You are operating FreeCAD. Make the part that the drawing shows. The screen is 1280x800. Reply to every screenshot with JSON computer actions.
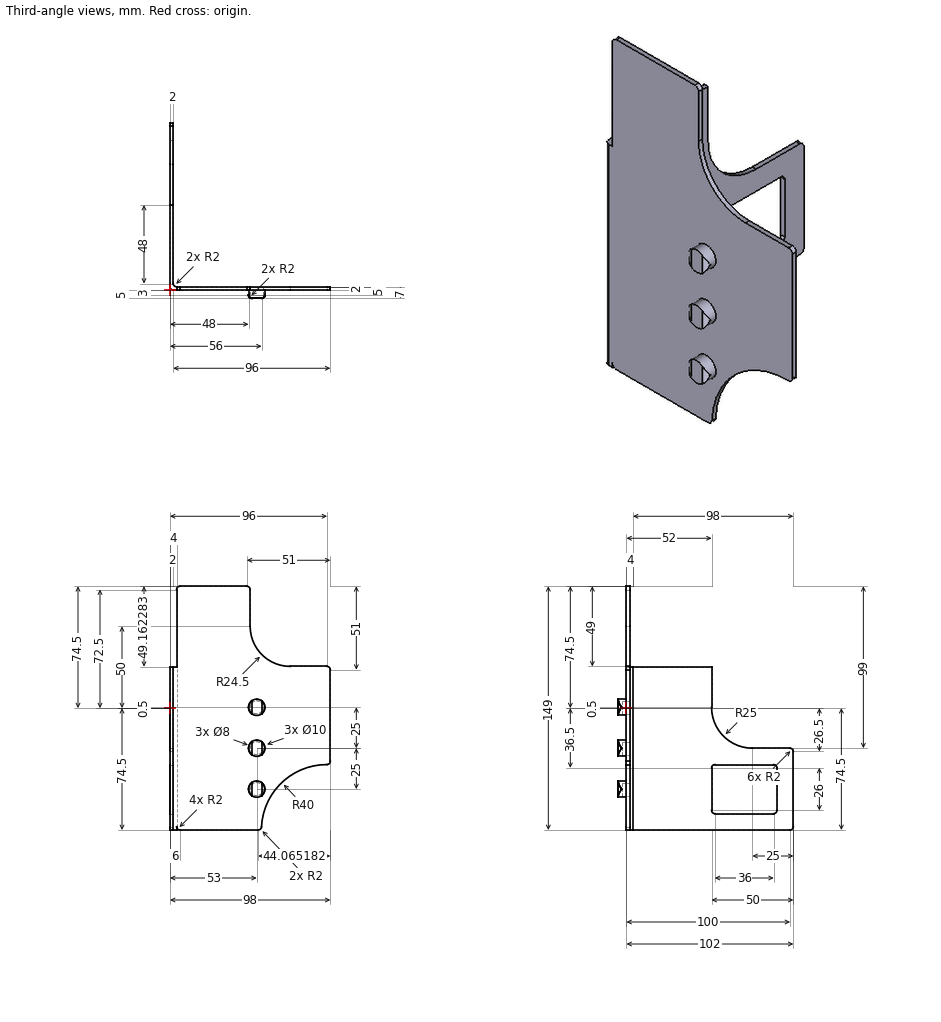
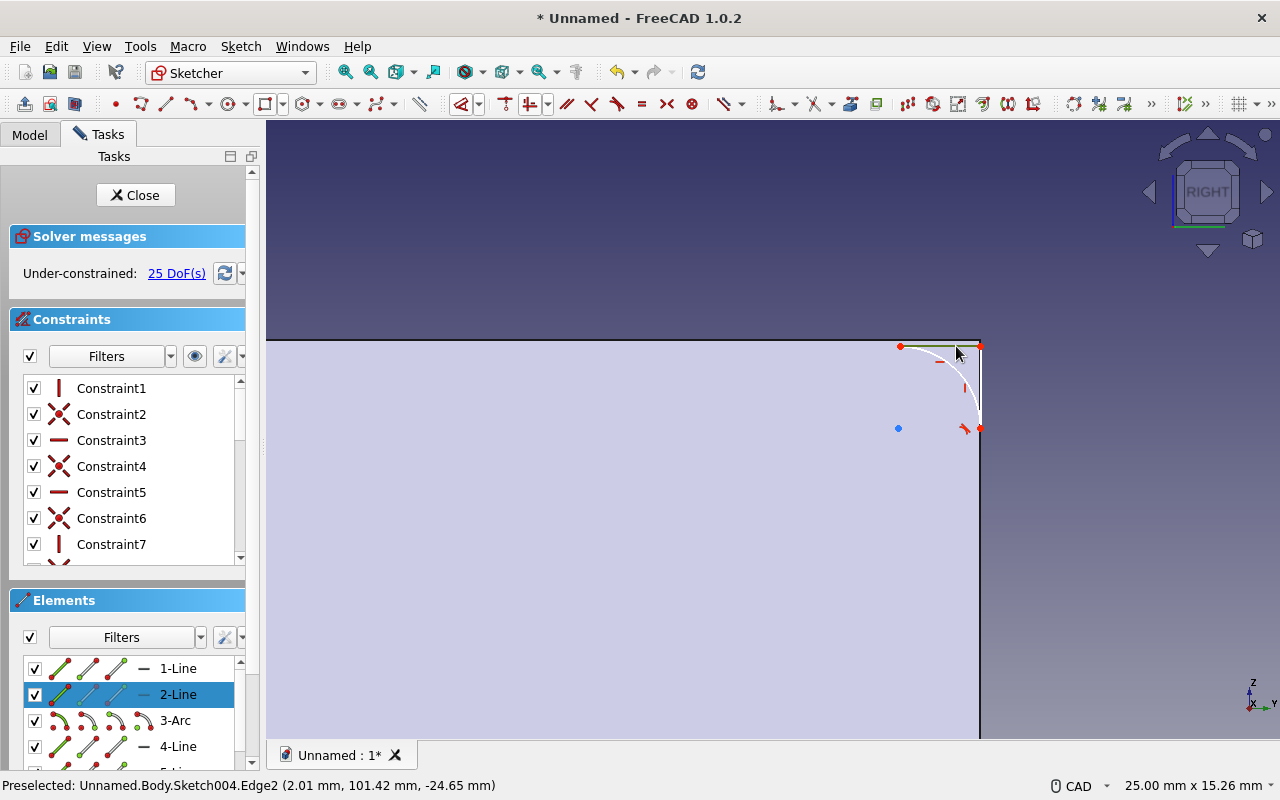
{"action": "scroll", "coordinate": [937, 356], "scroll_direction": "up", "scroll_amount": 3}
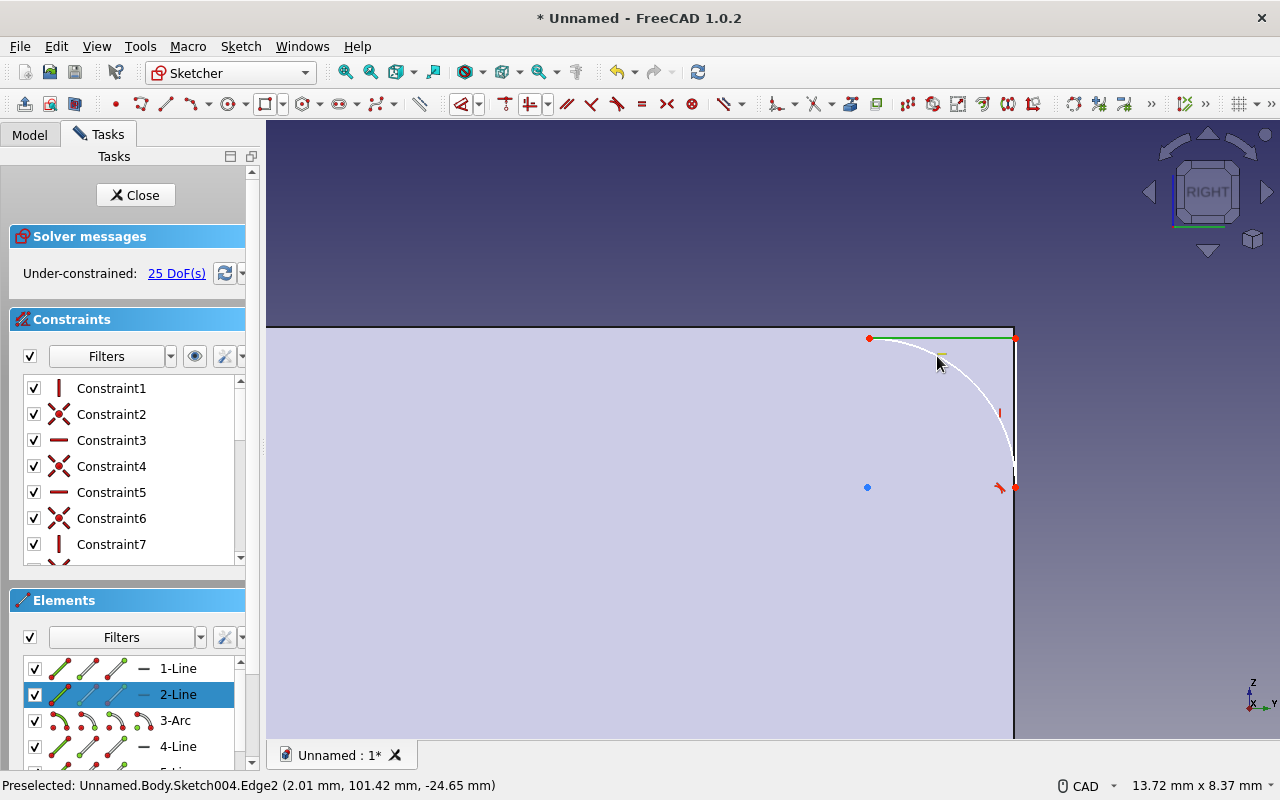
{"action": "left_click", "coordinate": [936, 355]}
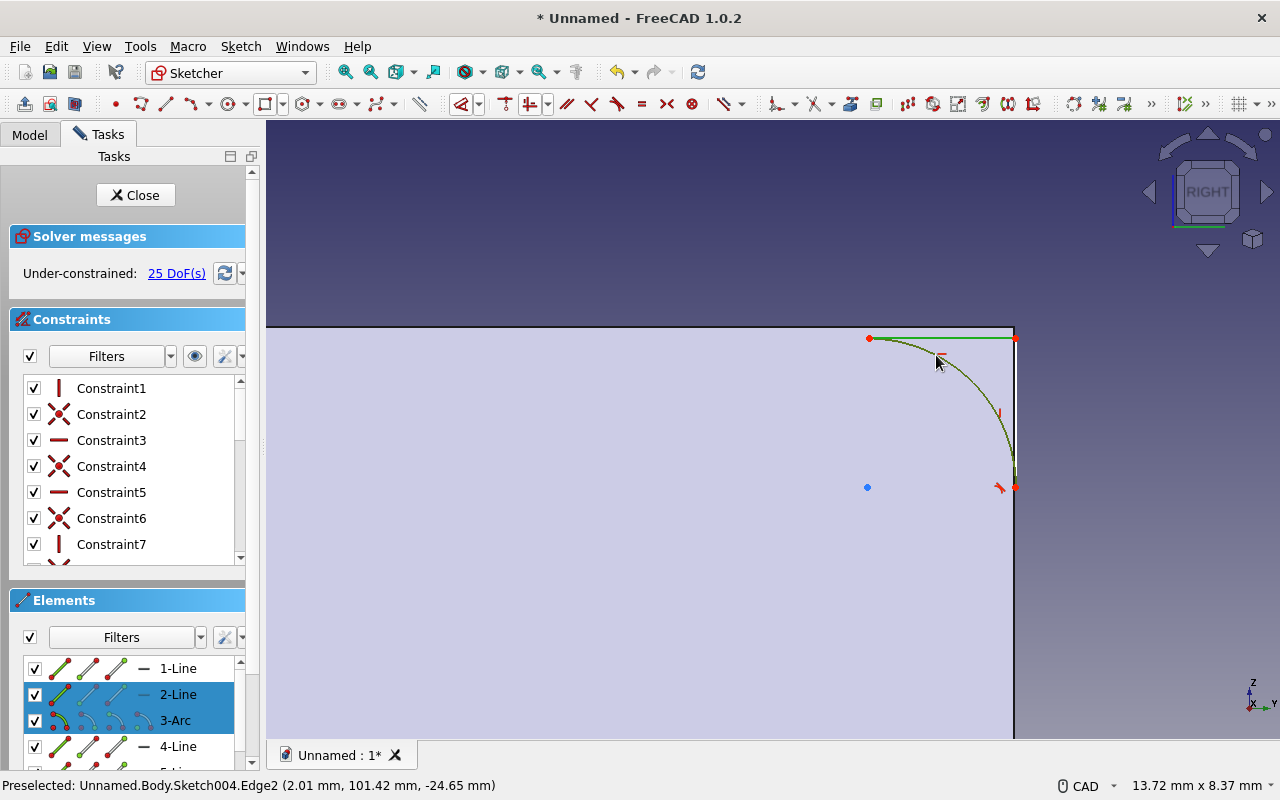
{"action": "key", "text": "t"}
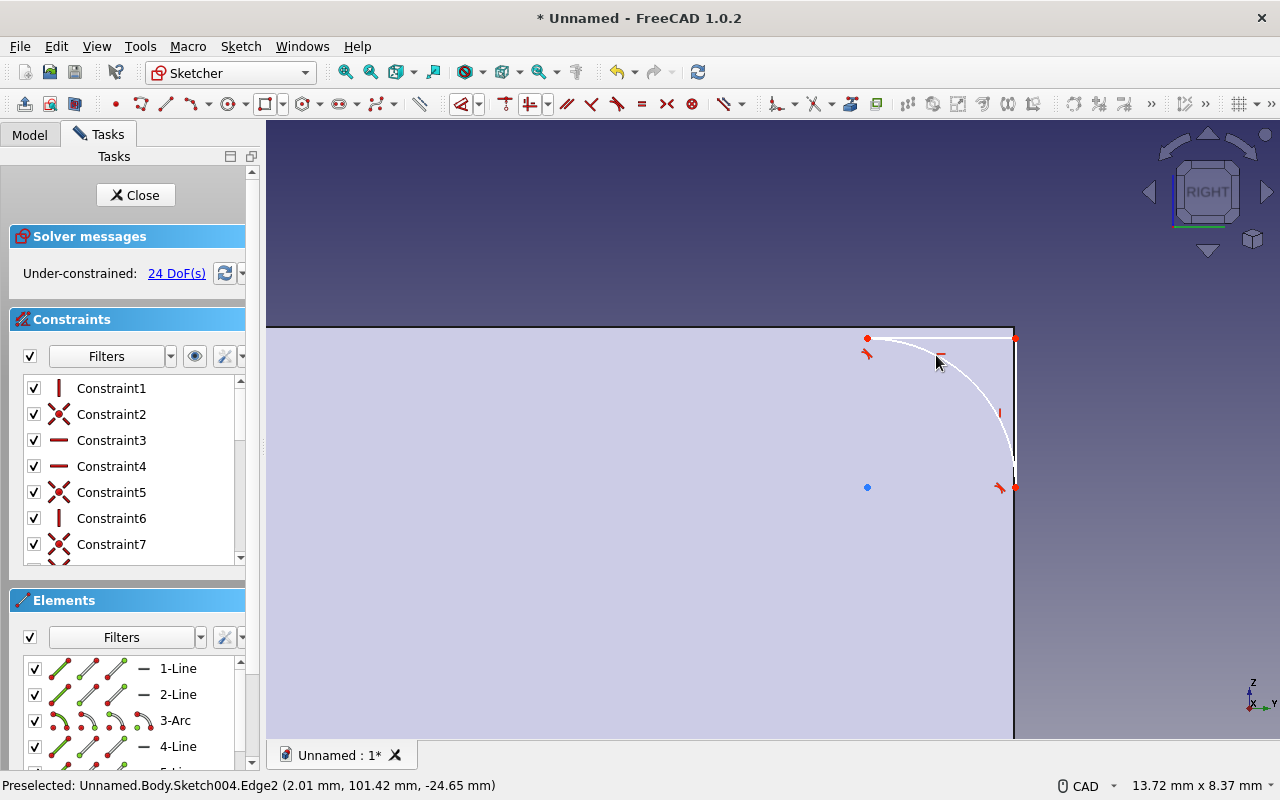
{"action": "scroll", "coordinate": [982, 362], "scroll_direction": "down", "scroll_amount": 13}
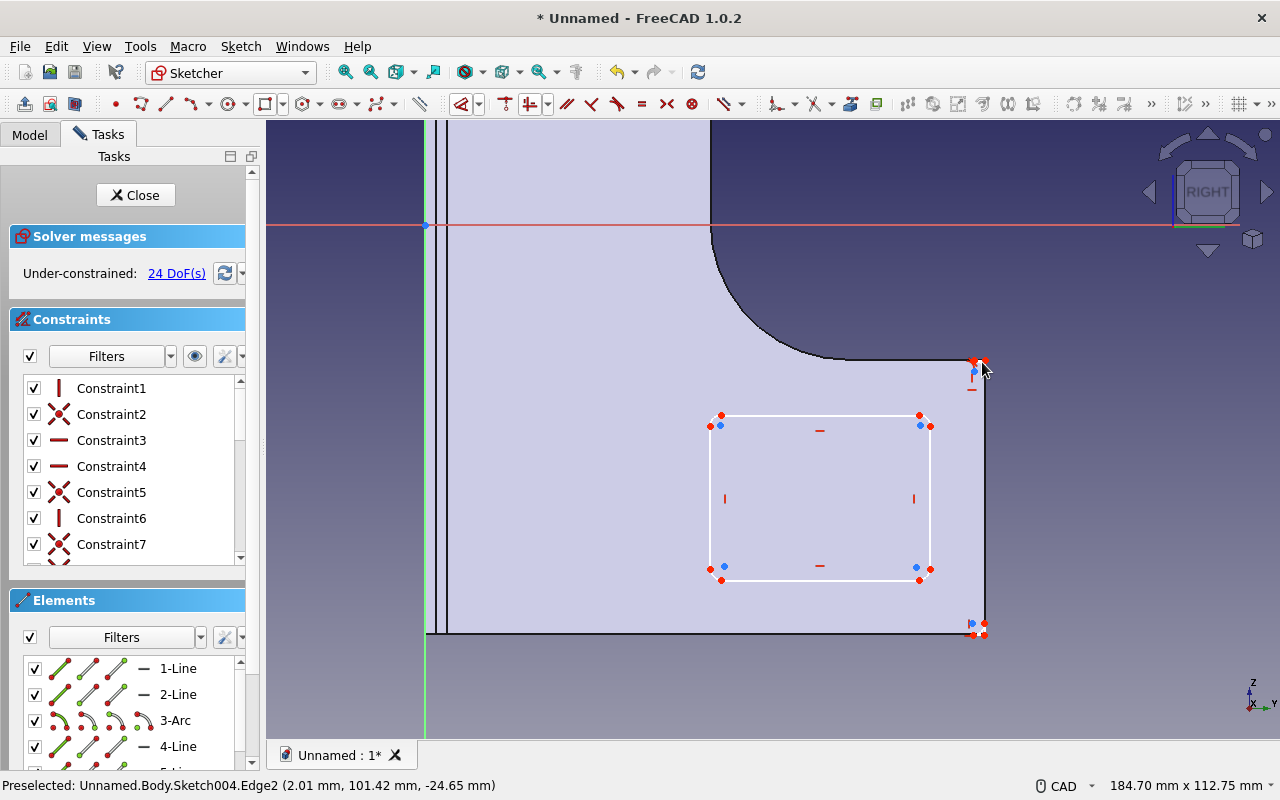
{"action": "scroll", "coordinate": [982, 635], "scroll_direction": "up", "scroll_amount": 9}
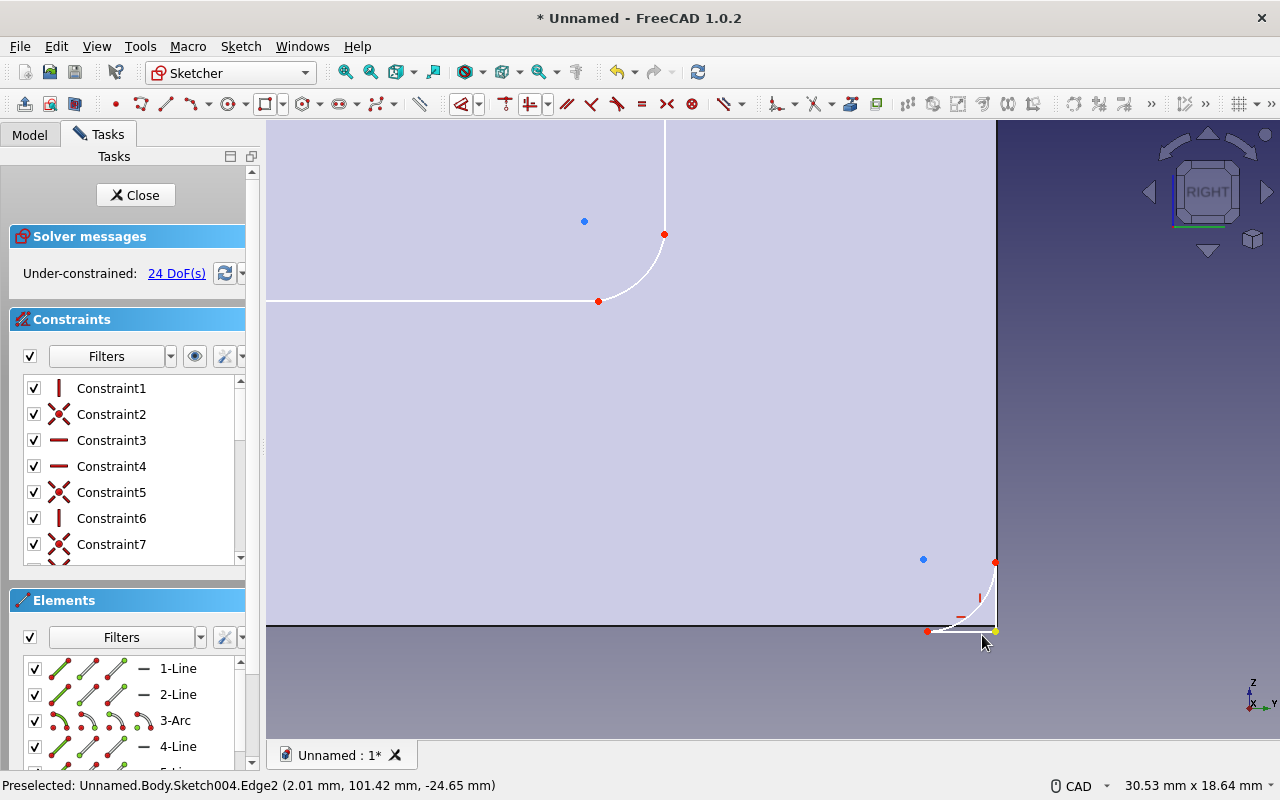
{"action": "left_click", "coordinate": [975, 632]}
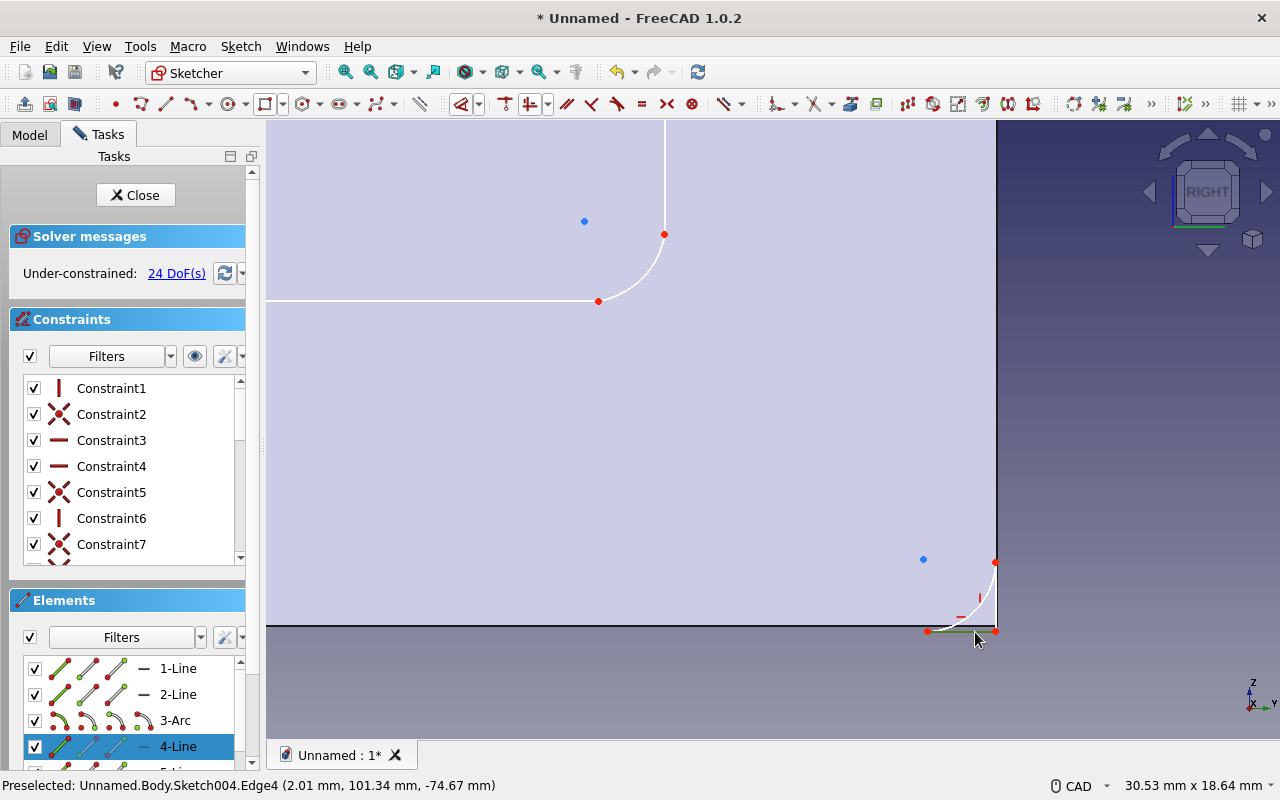
{"action": "left_click", "coordinate": [975, 610]}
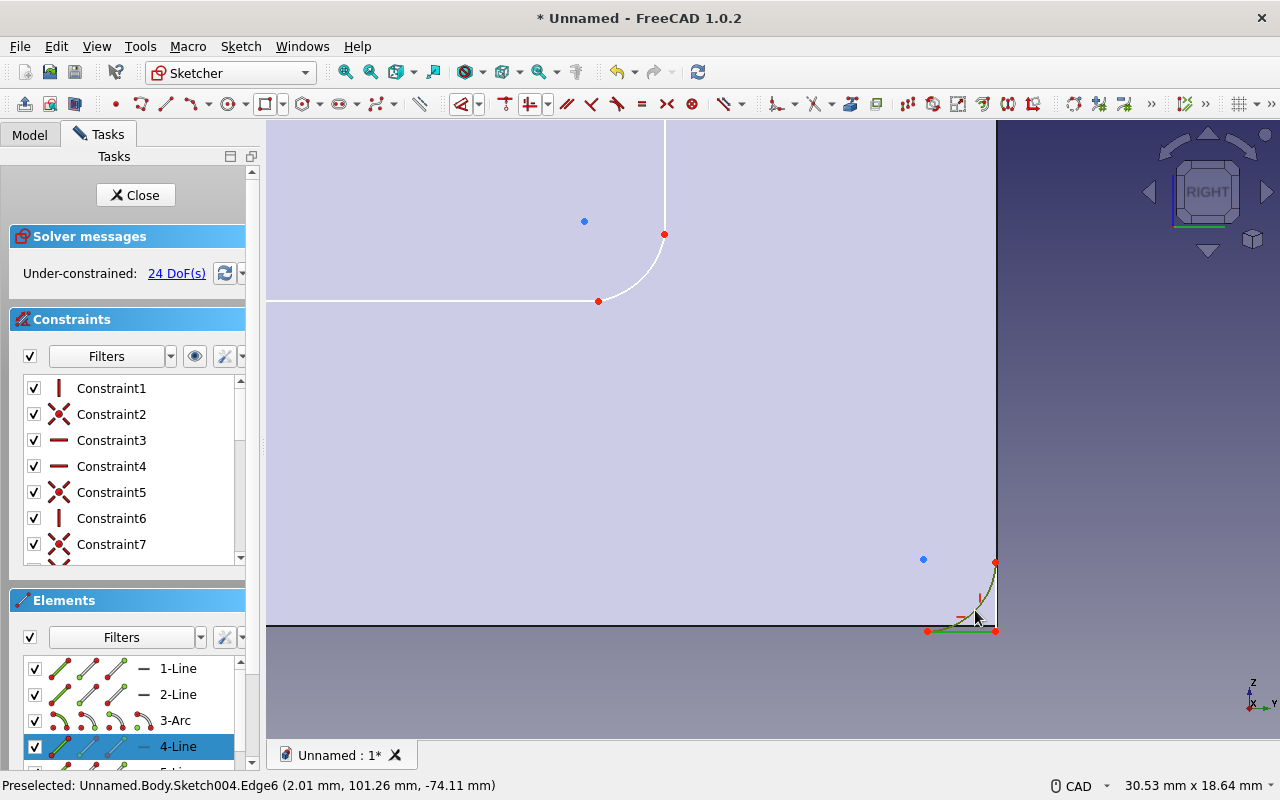
{"action": "key", "text": "t"}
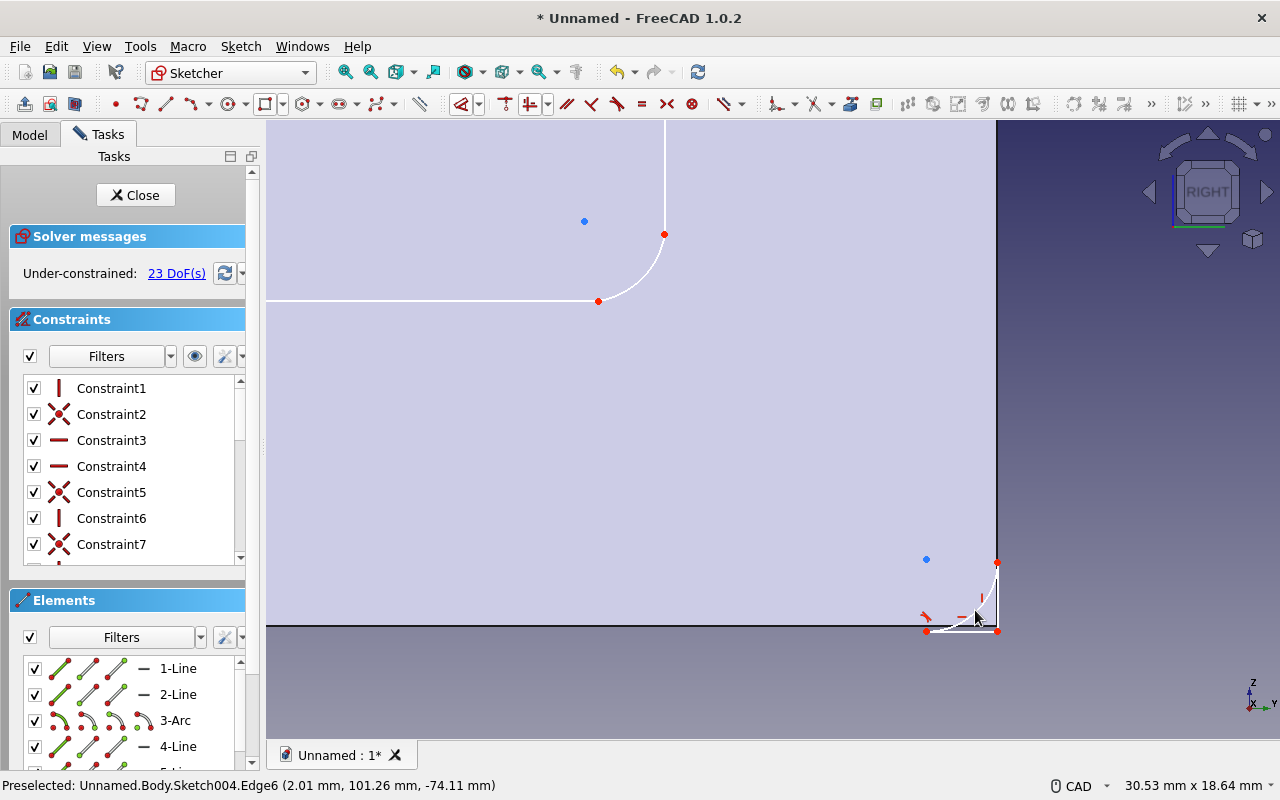
{"action": "left_click", "coordinate": [998, 611]}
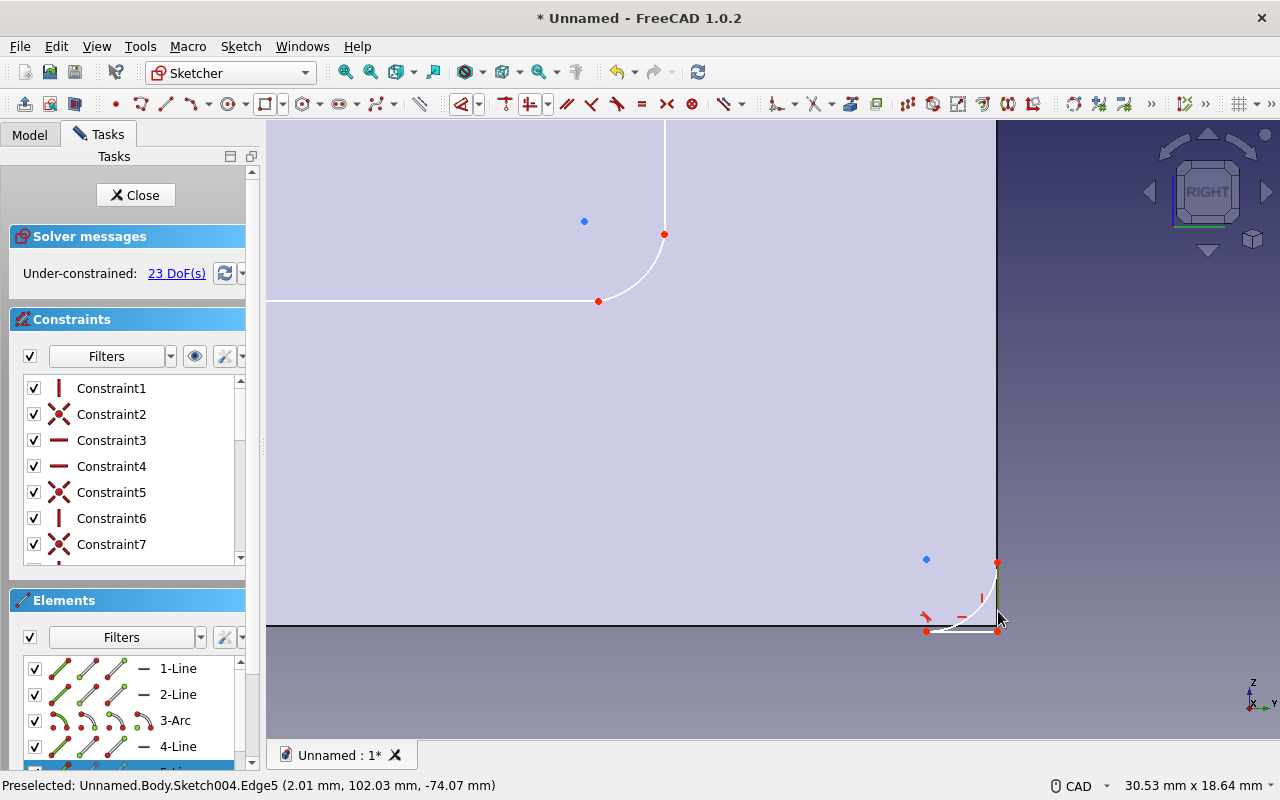
{"action": "left_click", "coordinate": [976, 612]}